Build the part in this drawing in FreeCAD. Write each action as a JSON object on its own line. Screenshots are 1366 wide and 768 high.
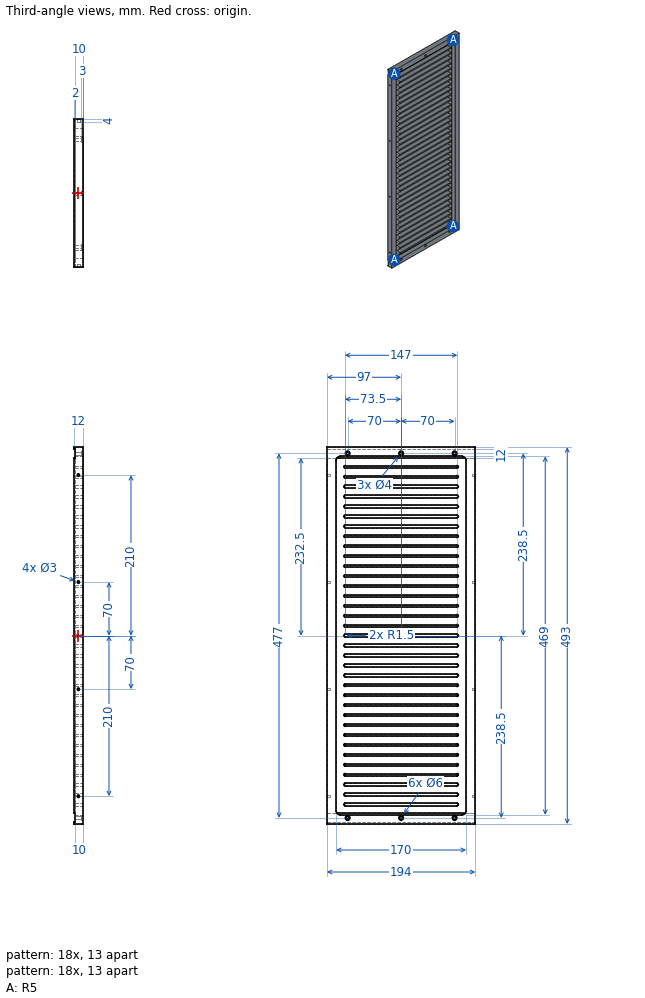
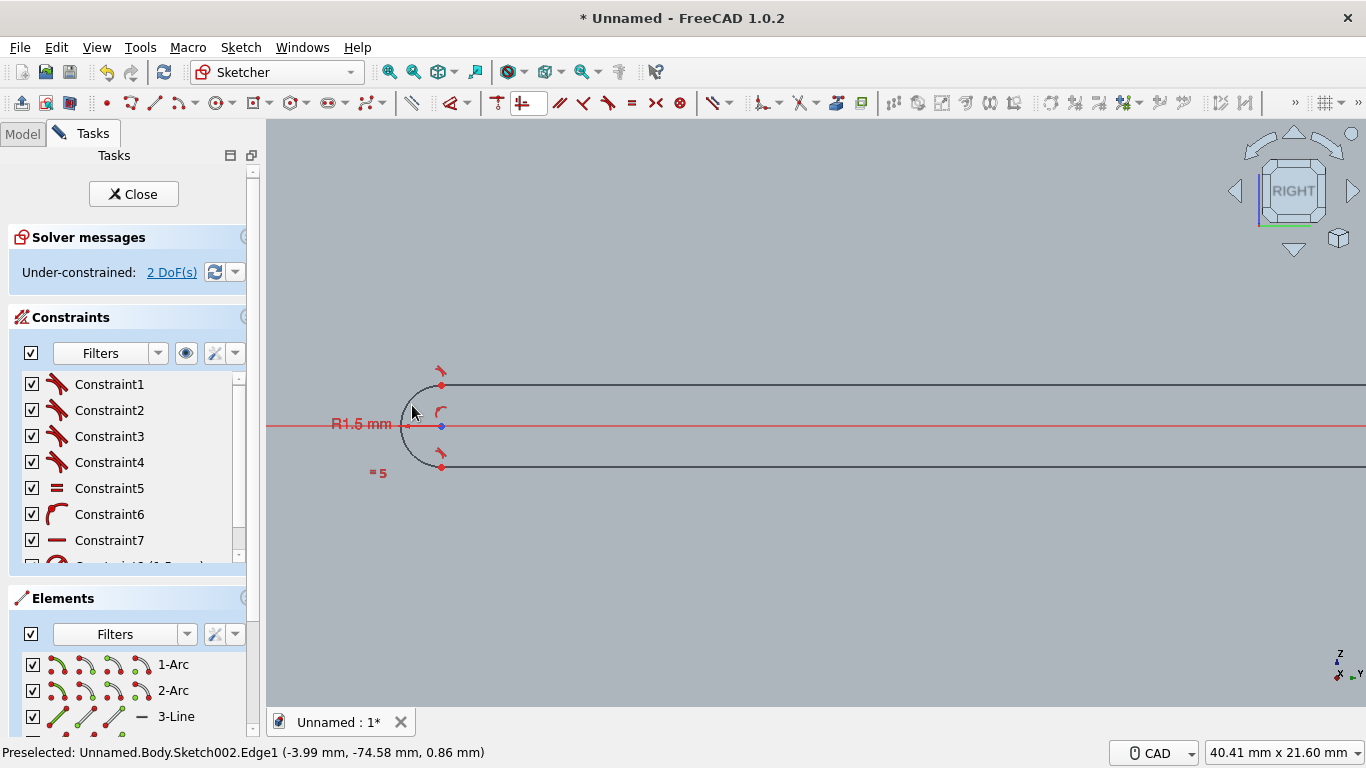
{"action": "scroll", "coordinate": [412, 410], "scroll_direction": "down", "scroll_amount": 9}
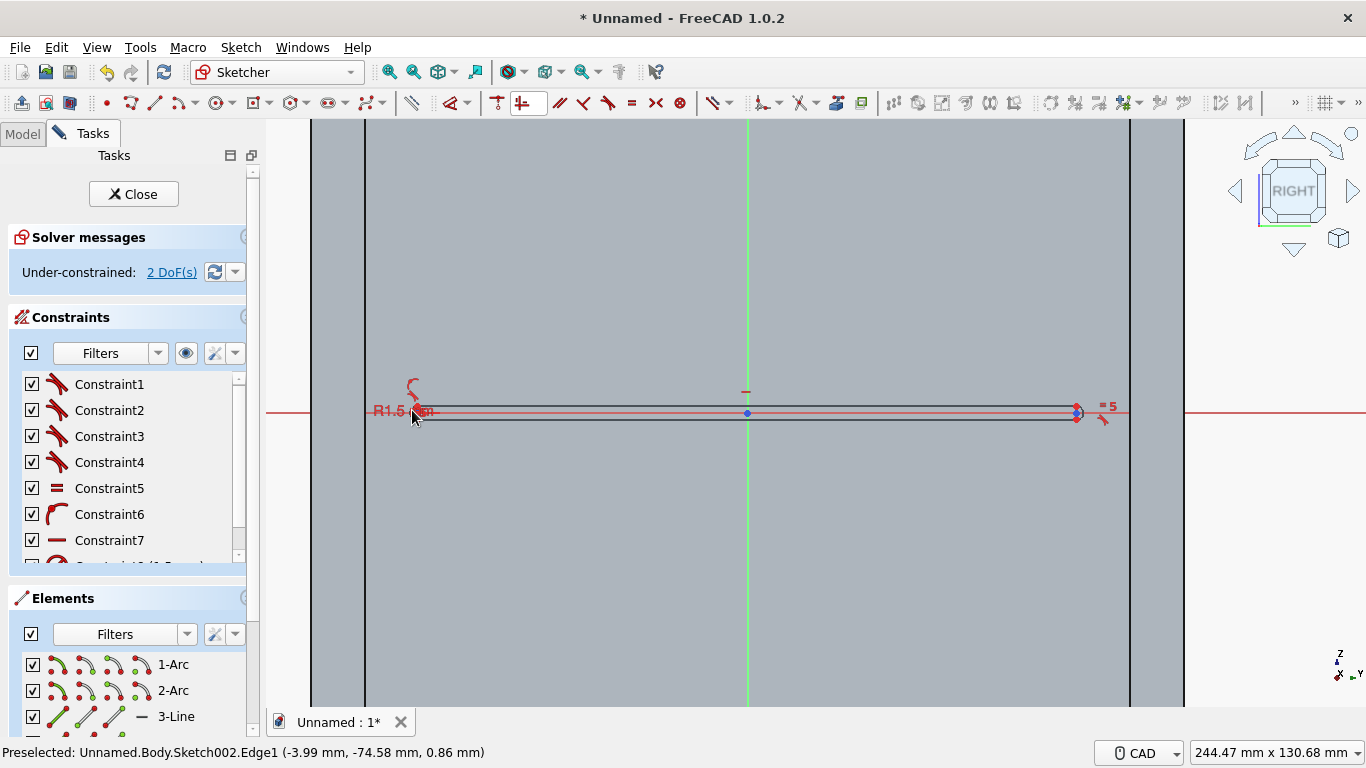
{"action": "scroll", "coordinate": [615, 406], "scroll_direction": "up", "scroll_amount": 4}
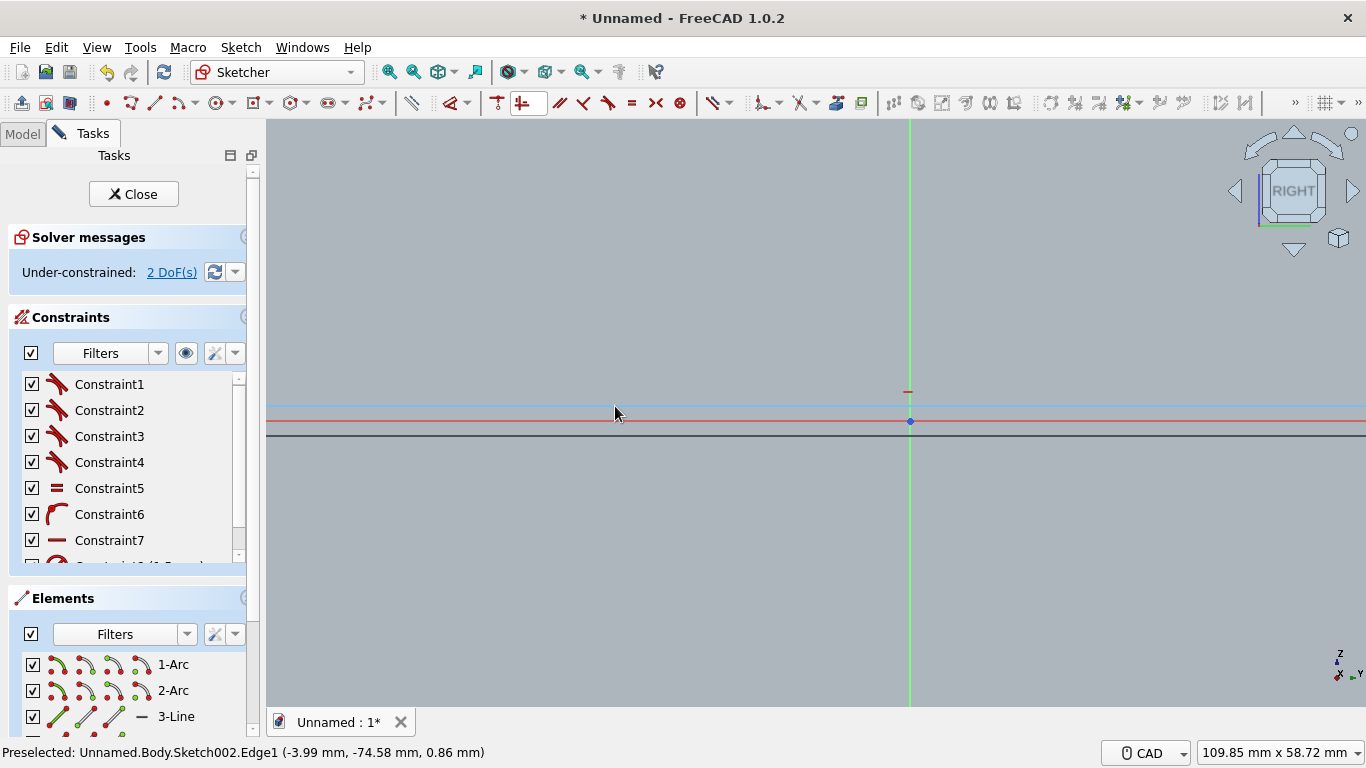
{"action": "left_click", "coordinate": [614, 406]}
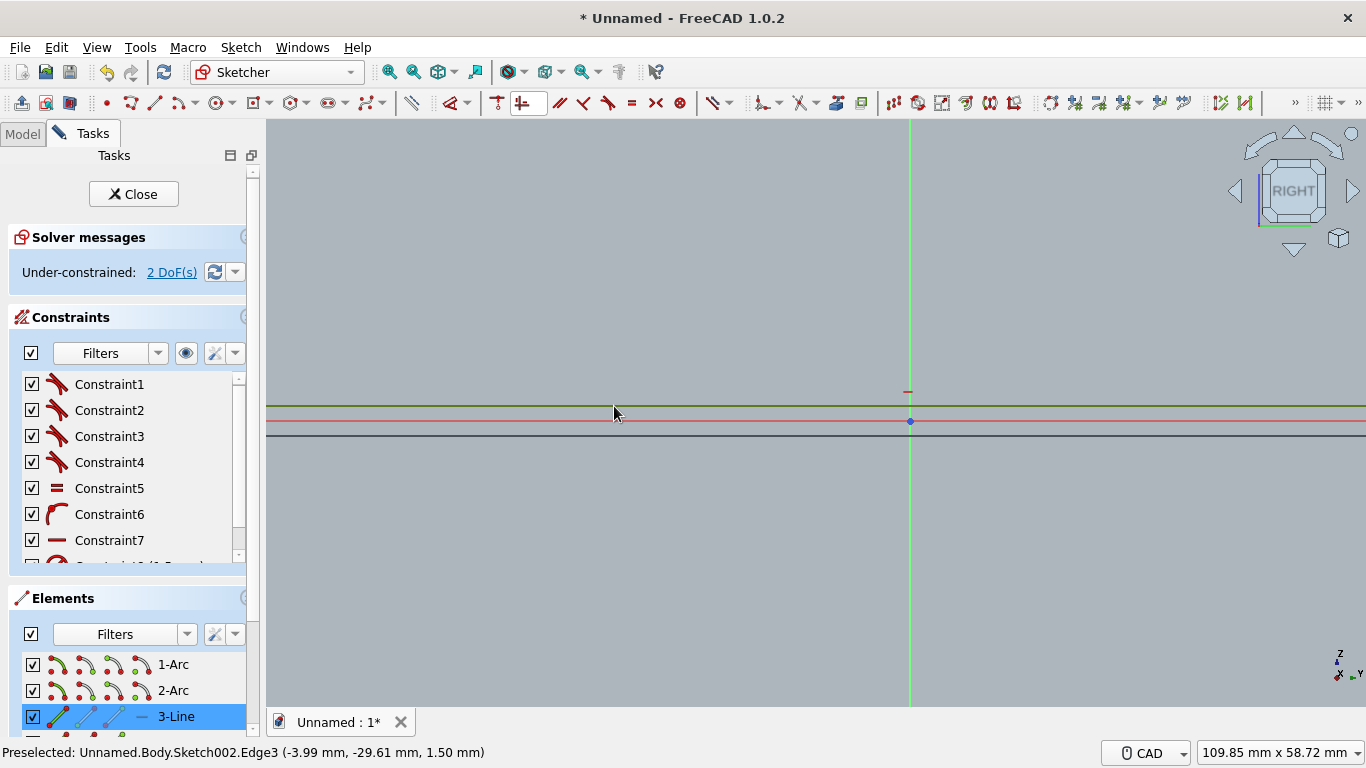
{"action": "key", "text": "l"}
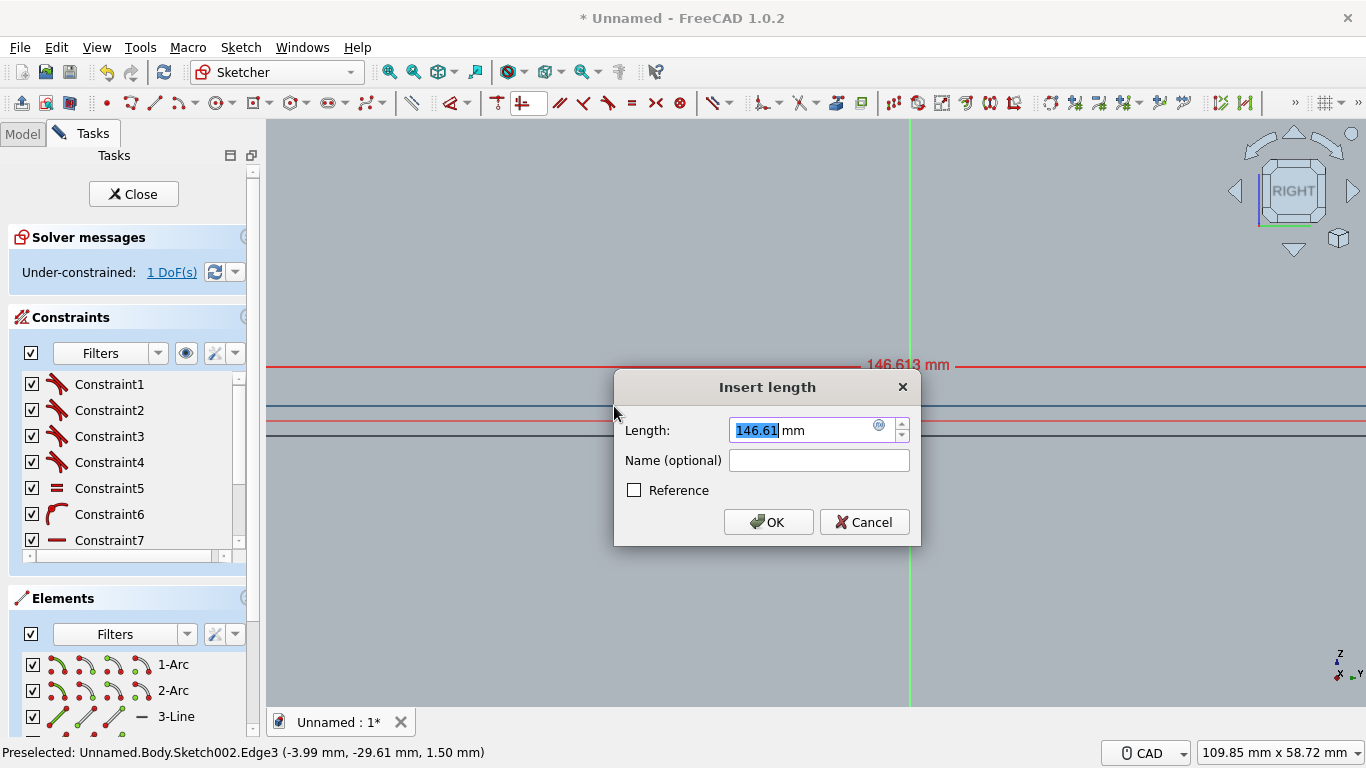
{"action": "type", "text": "147"}
{"action": "key", "text": "Return"}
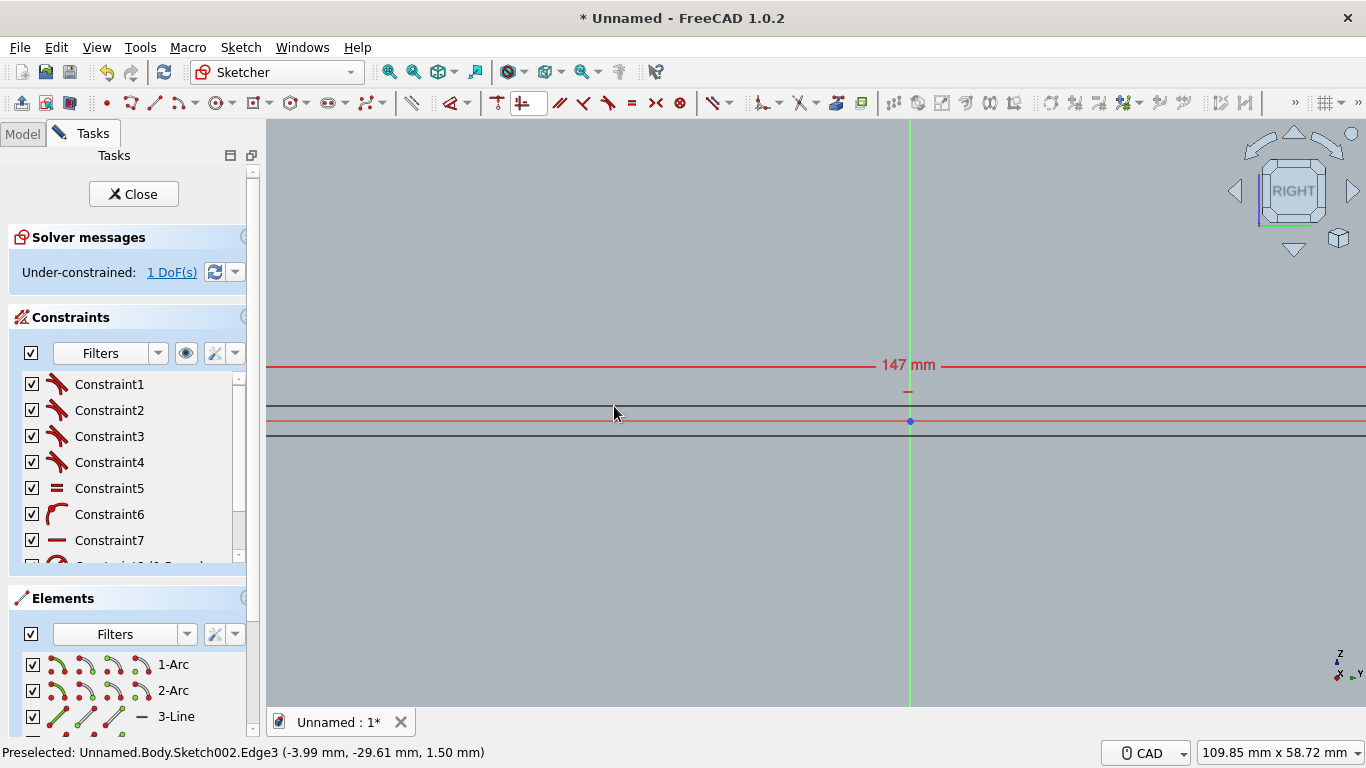
{"action": "scroll", "coordinate": [615, 406], "scroll_direction": "down", "scroll_amount": 4}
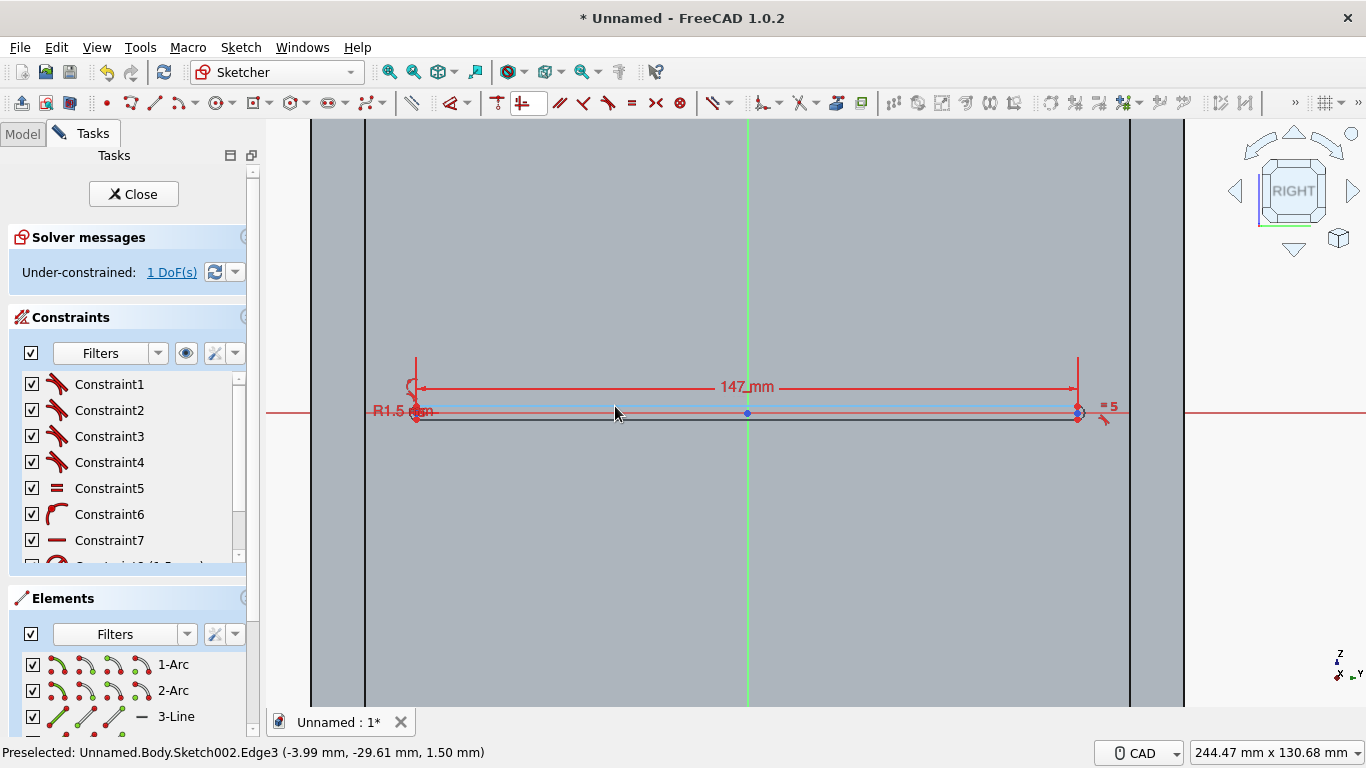
{"action": "scroll", "coordinate": [416, 406], "scroll_direction": "up", "scroll_amount": 3}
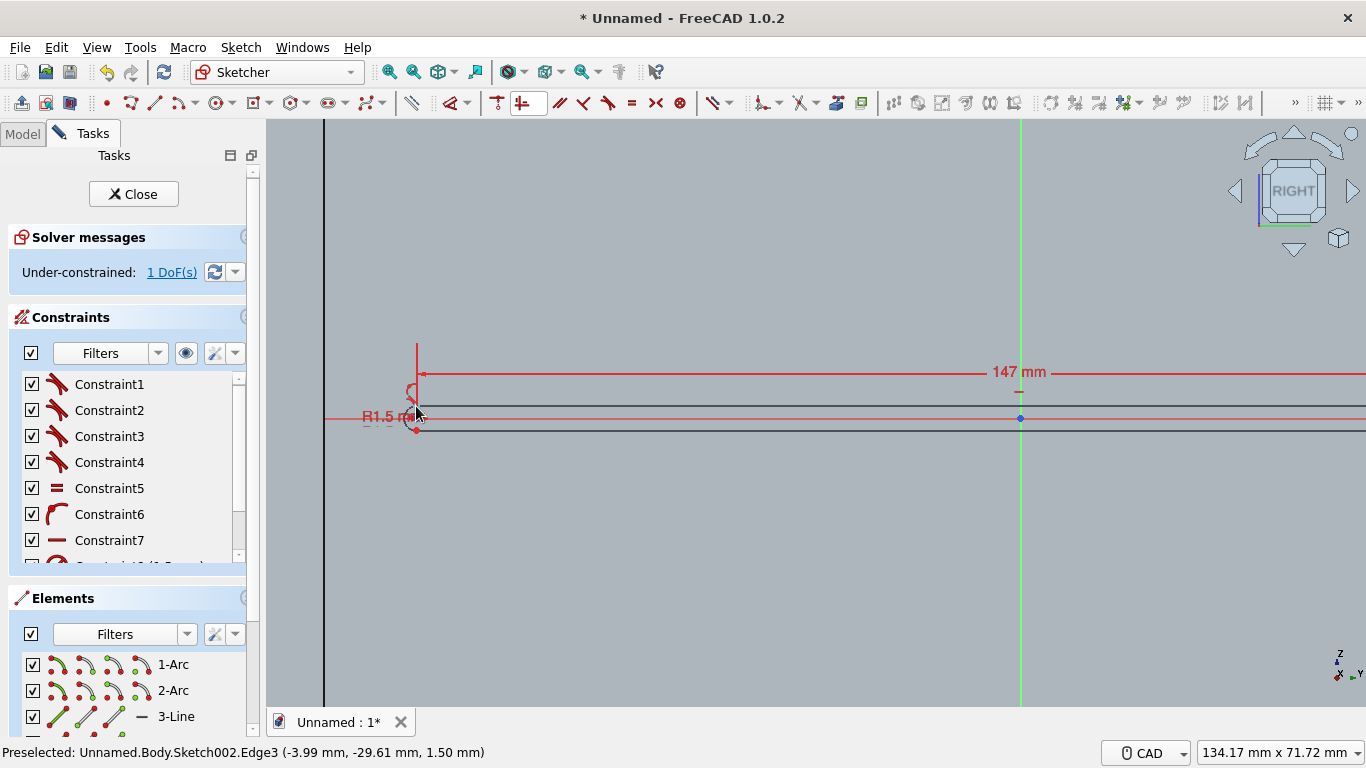
{"action": "left_click", "coordinate": [417, 406]}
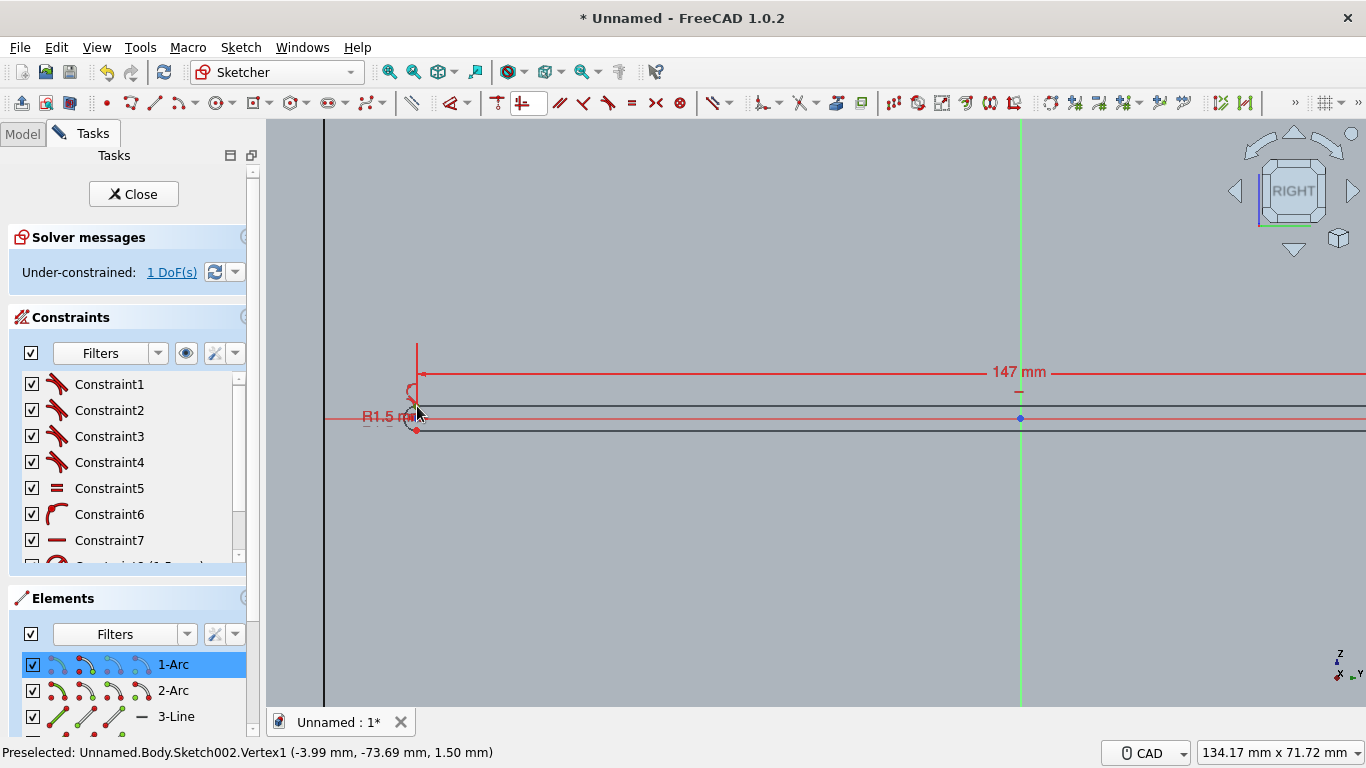
{"action": "key", "text": "l"}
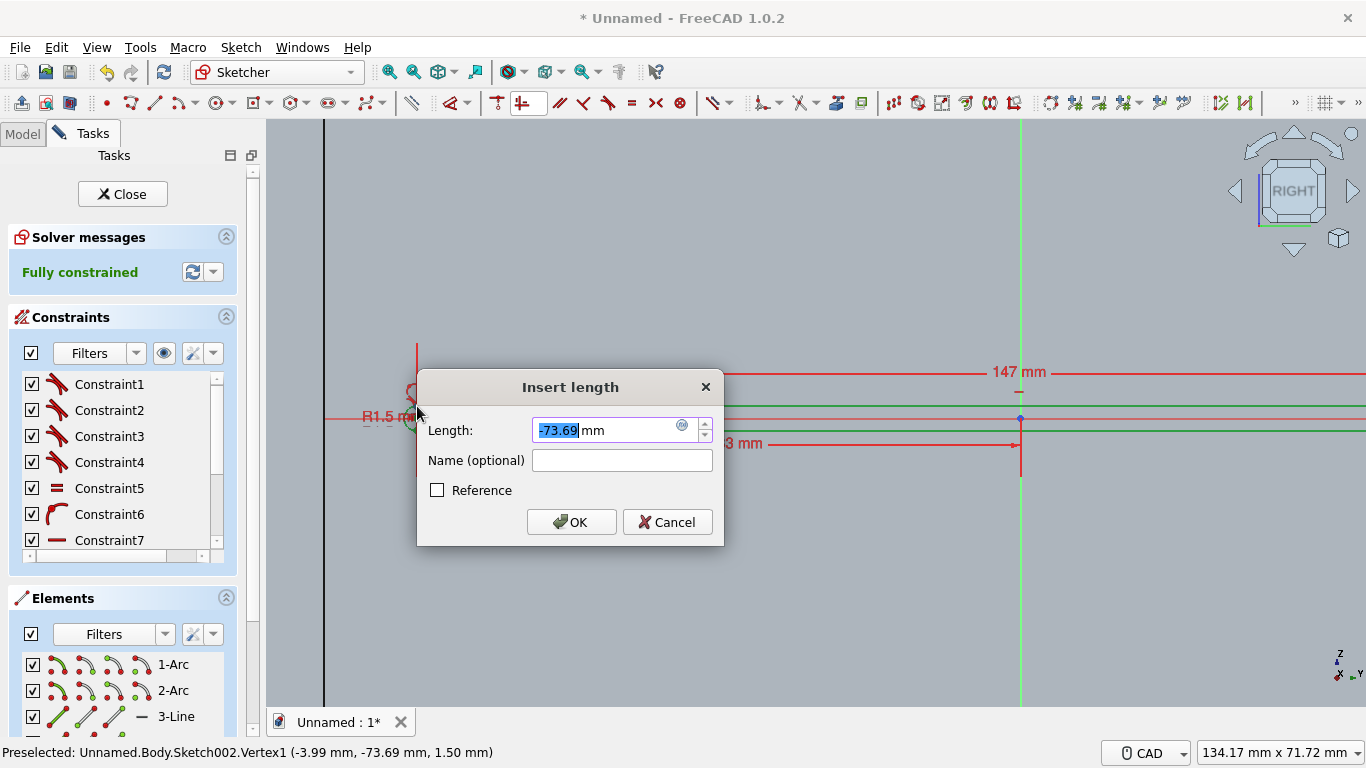
{"action": "type", "text": "-73.5"}
{"action": "key", "text": "Return"}